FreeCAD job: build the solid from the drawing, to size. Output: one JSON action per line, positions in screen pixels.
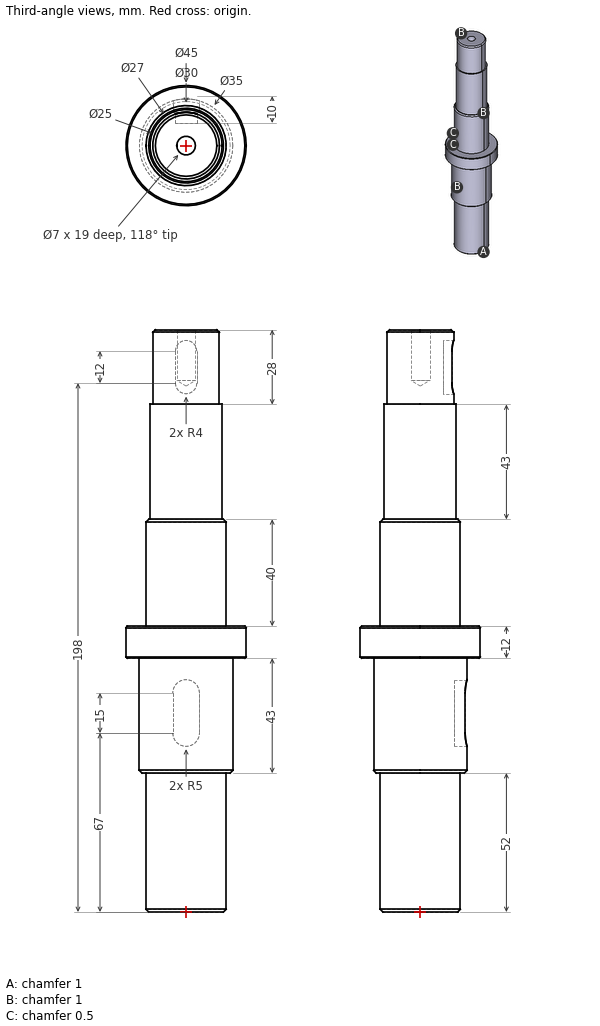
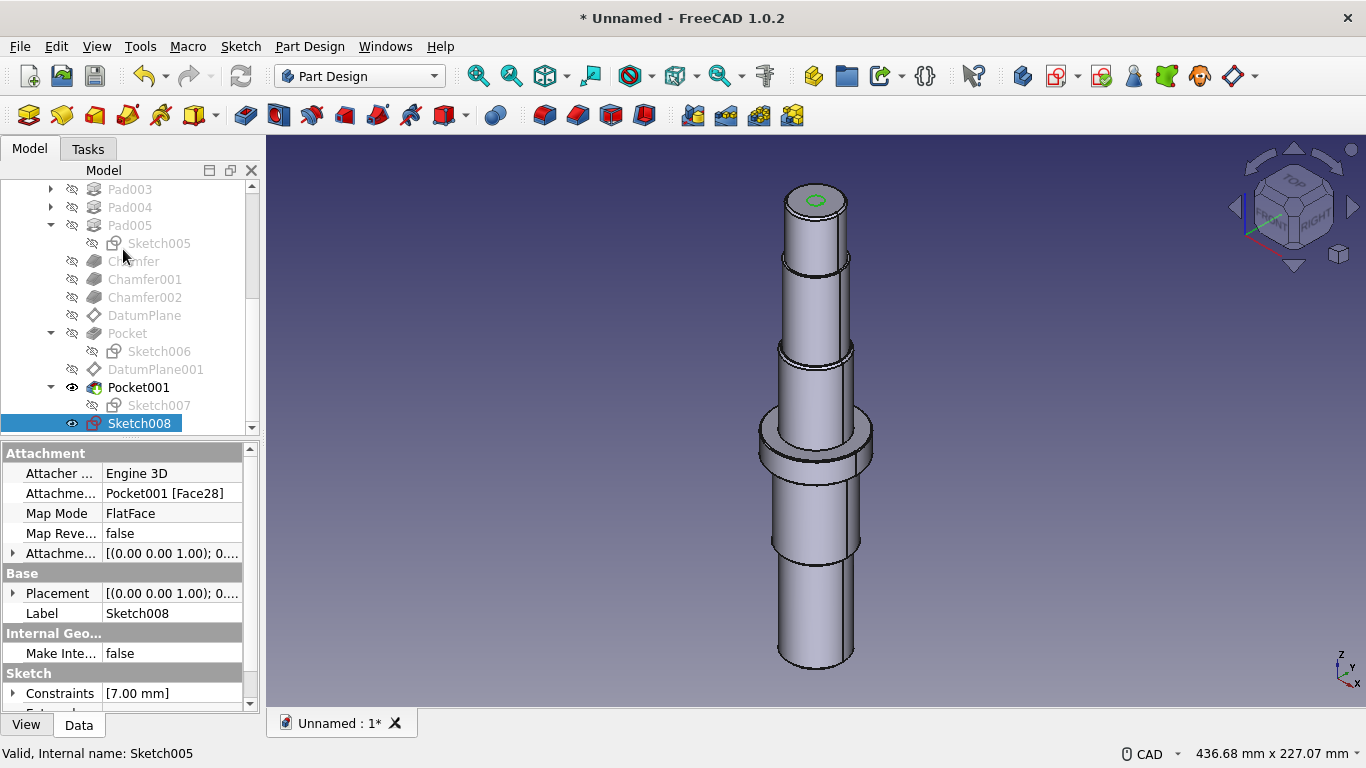
{"action": "left_click", "coordinate": [279, 116]}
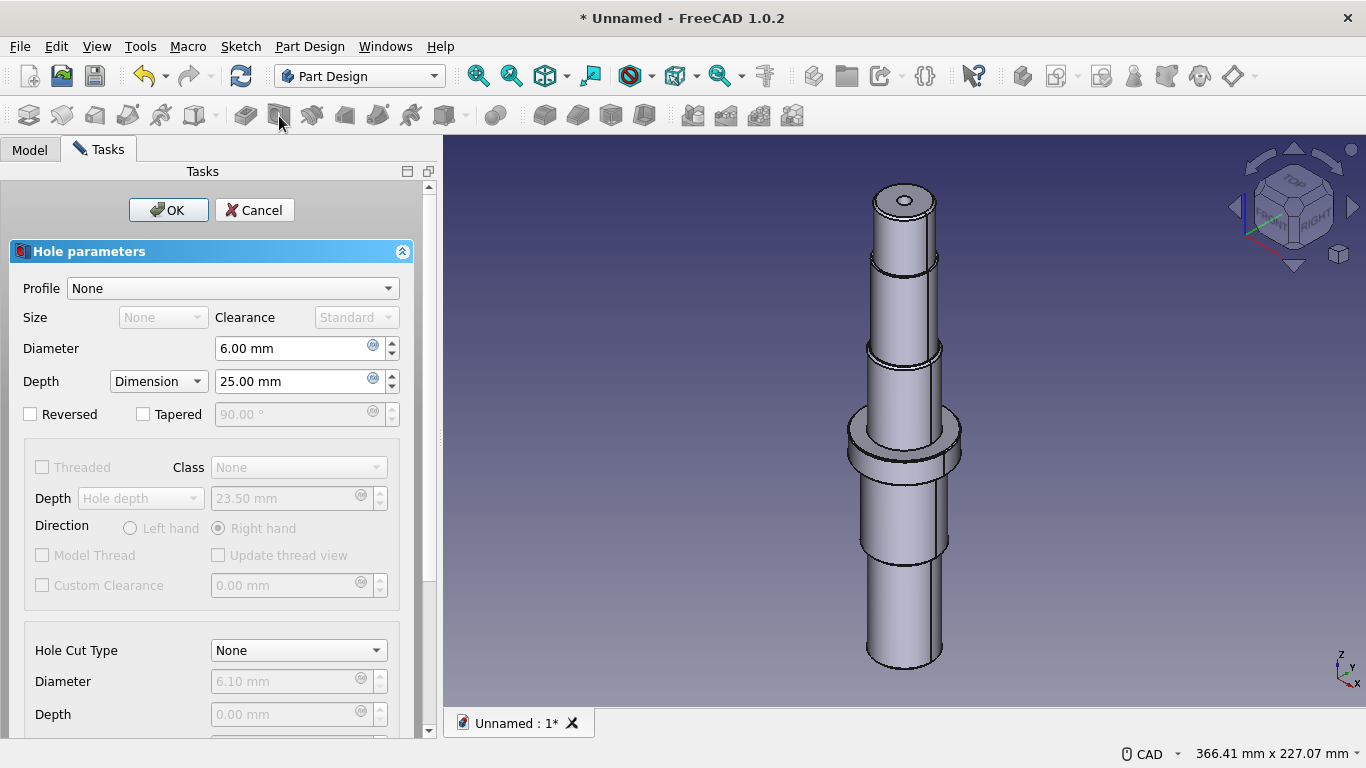
{"action": "triple_click", "coordinate": [300, 348]}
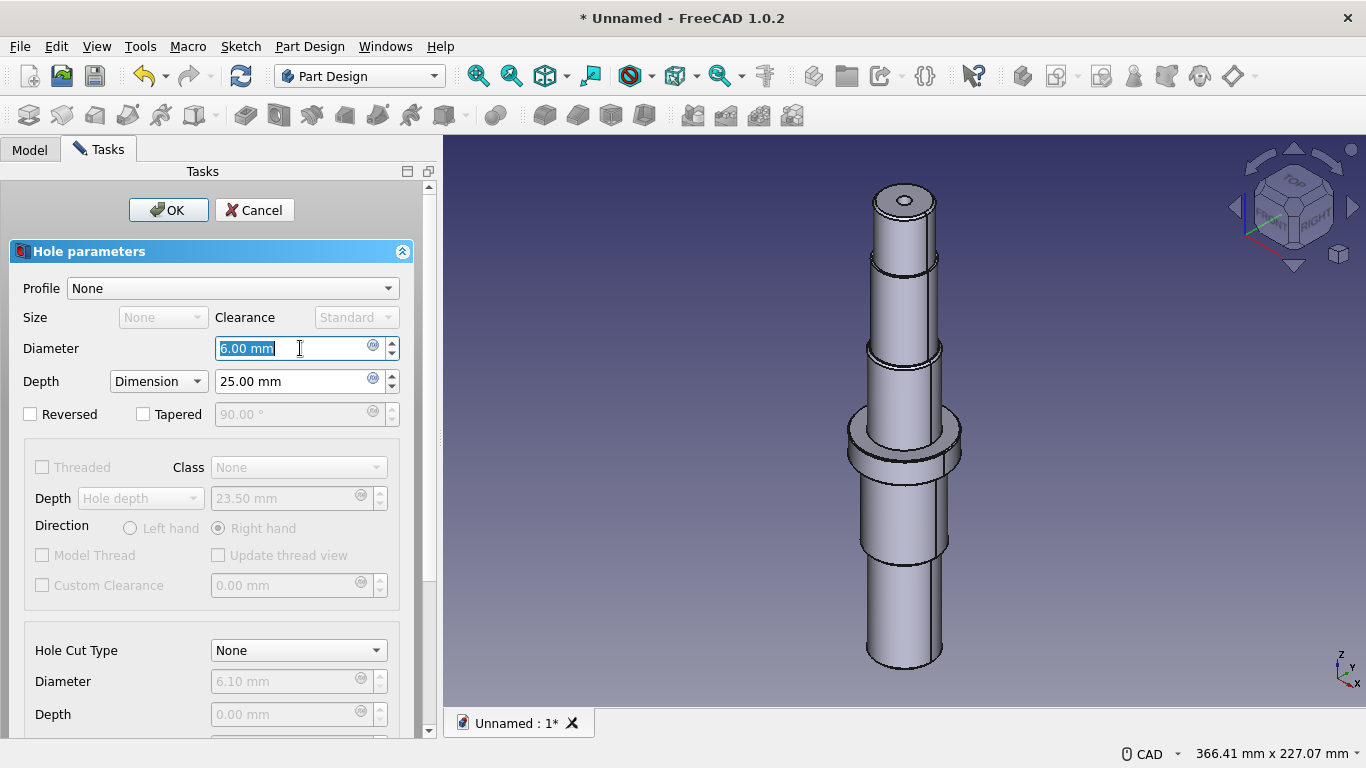
{"action": "type", "text": "7"}
{"action": "key", "text": "Tab"}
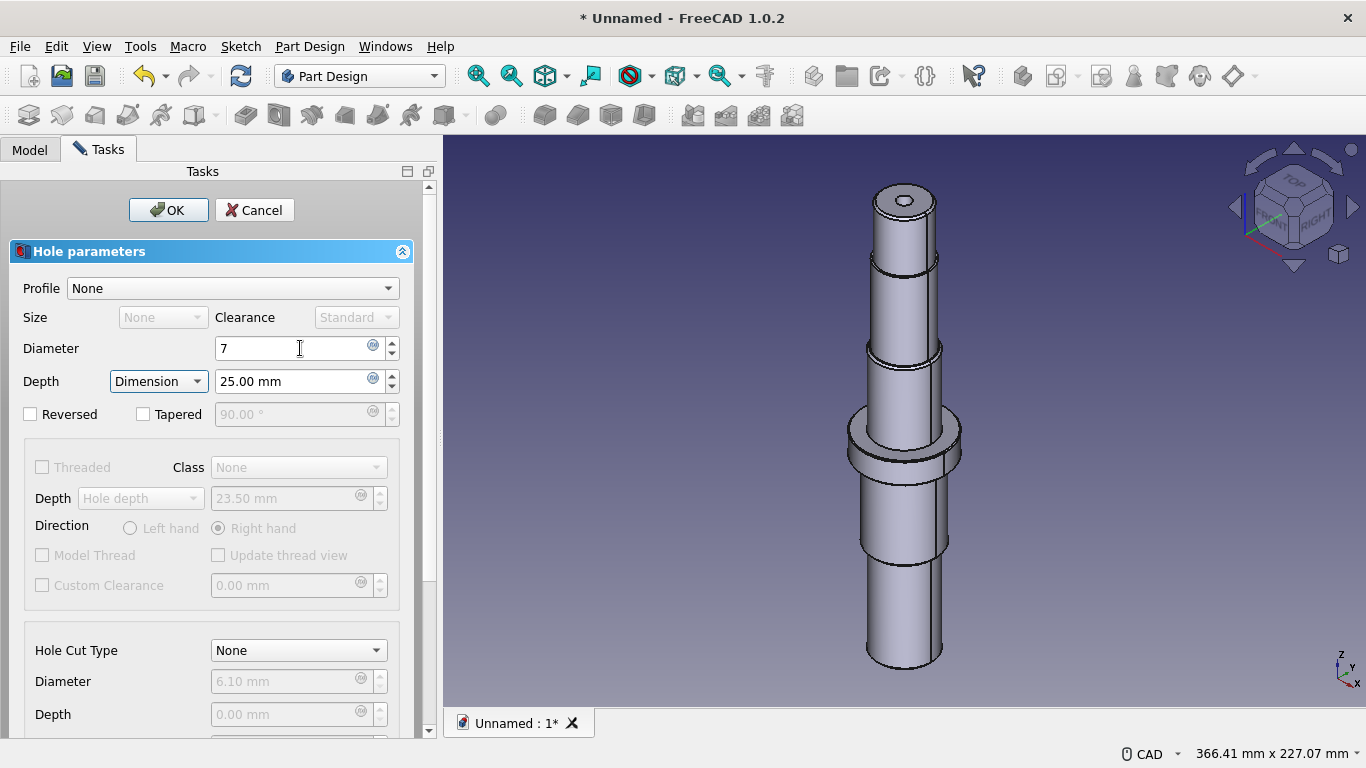
{"action": "triple_click", "coordinate": [300, 382]}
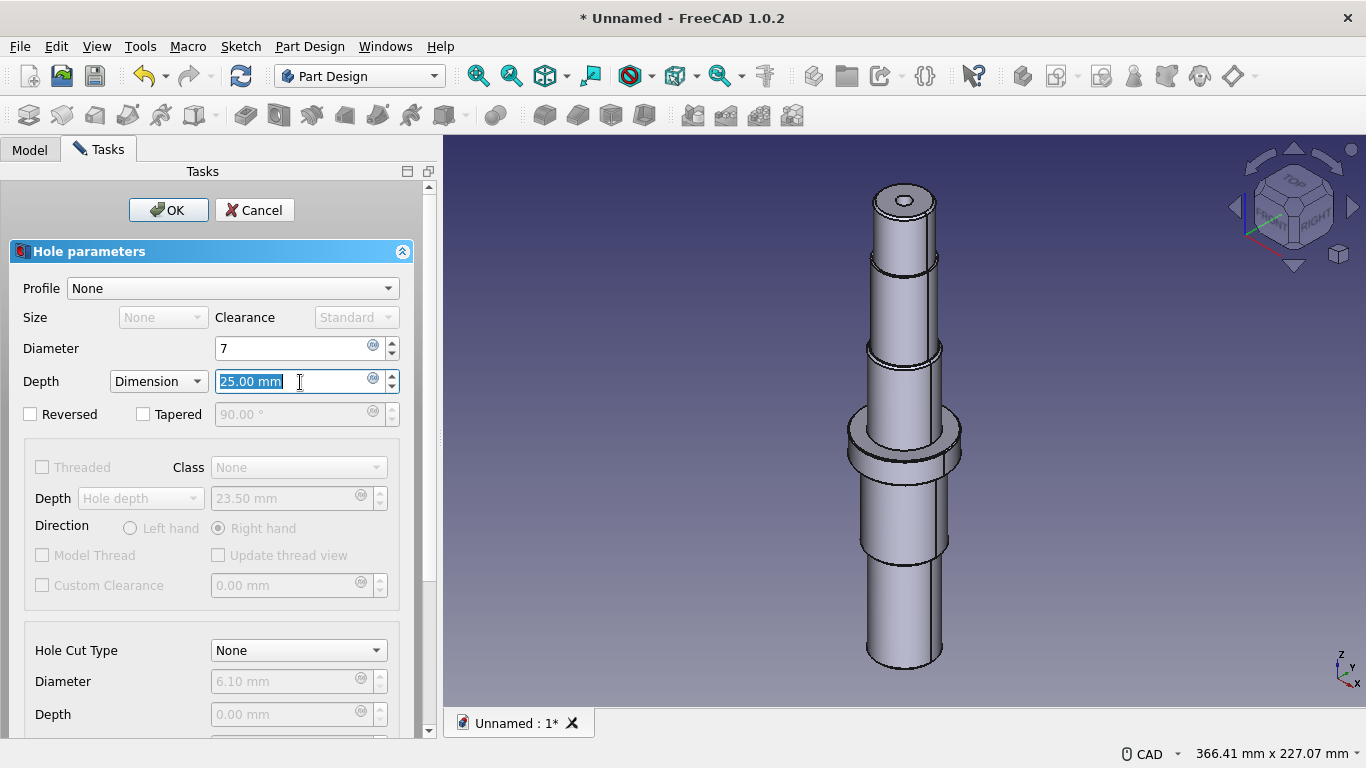
{"action": "type", "text": "19"}
{"action": "key", "text": "Tab"}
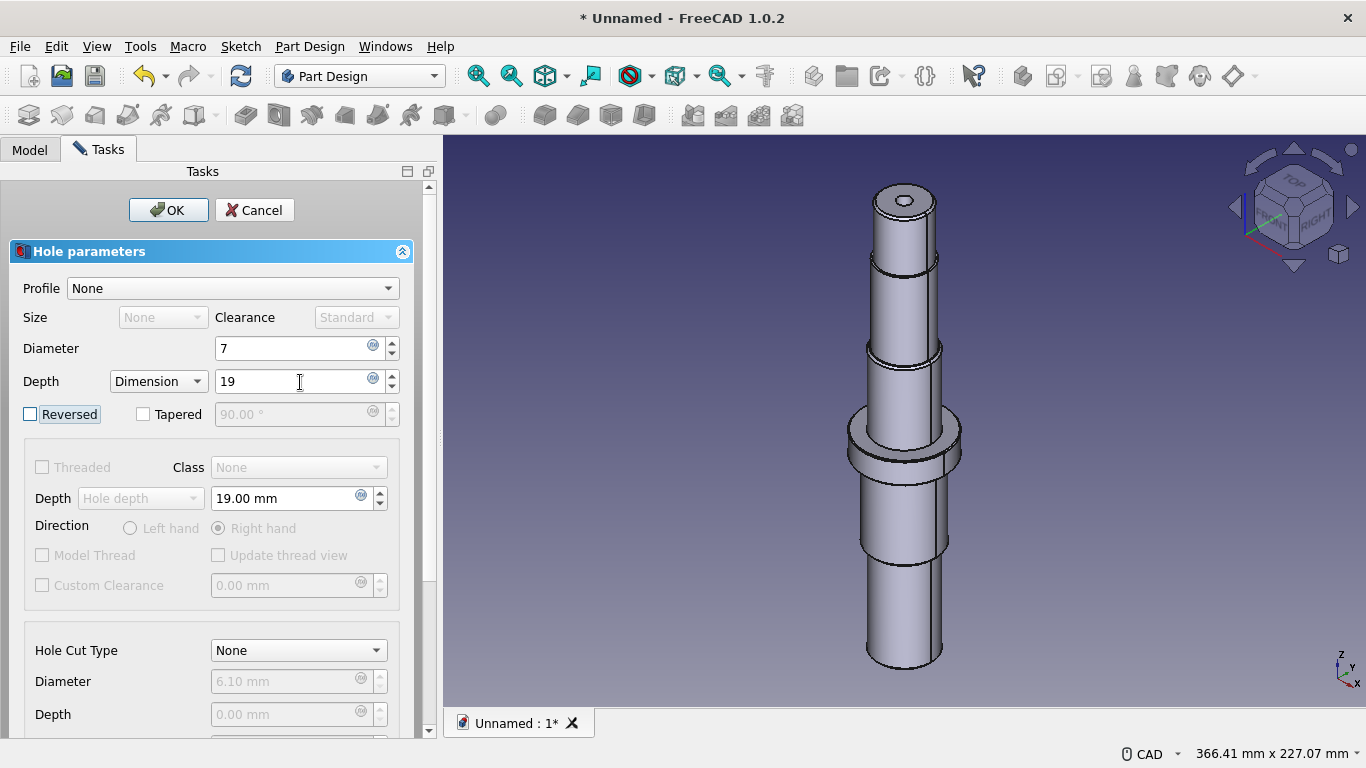
{"action": "left_click", "coordinate": [169, 210]}